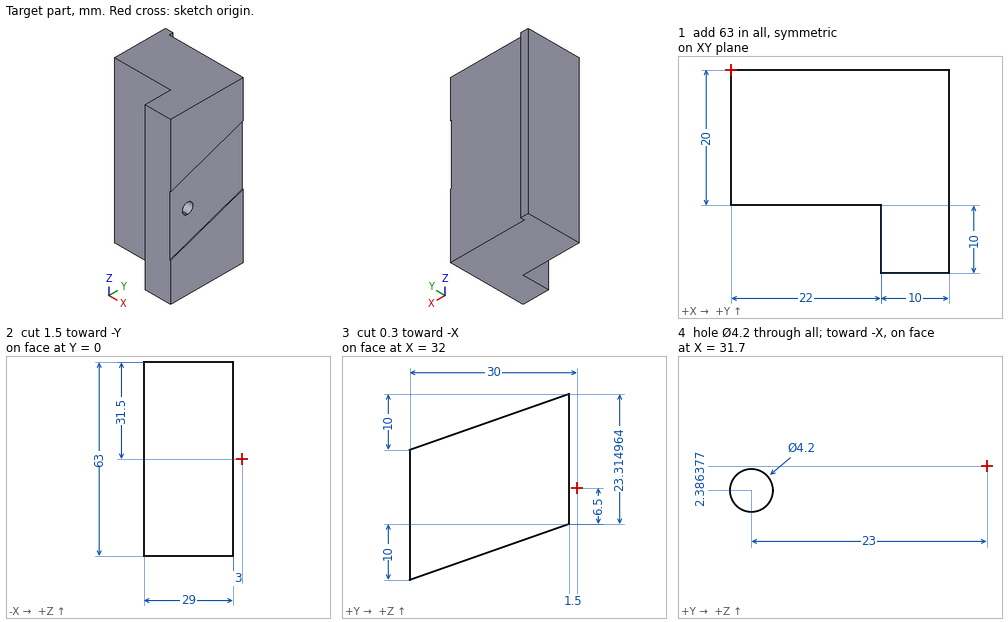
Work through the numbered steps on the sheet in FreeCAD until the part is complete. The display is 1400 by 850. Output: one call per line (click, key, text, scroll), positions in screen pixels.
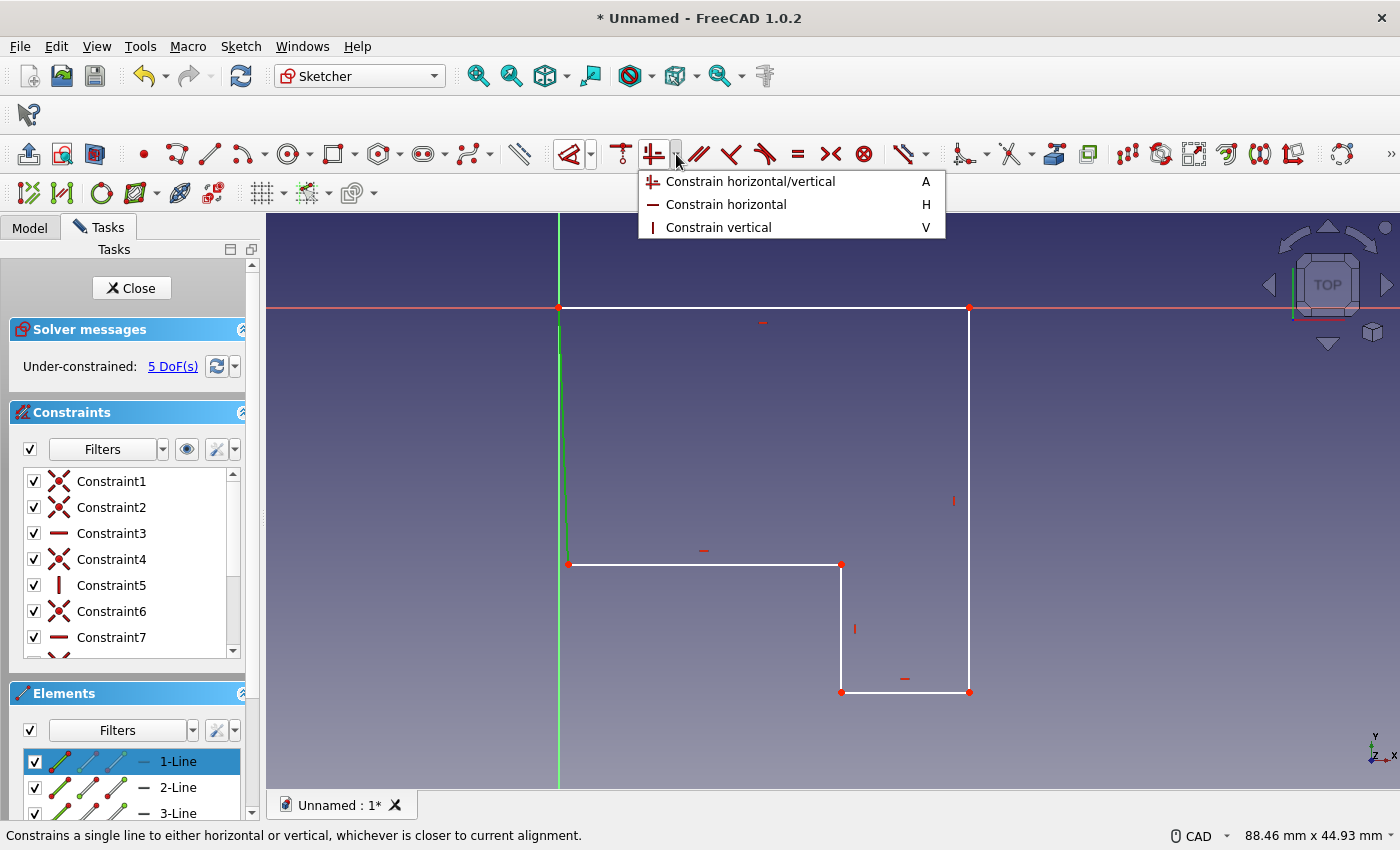
click(792, 228)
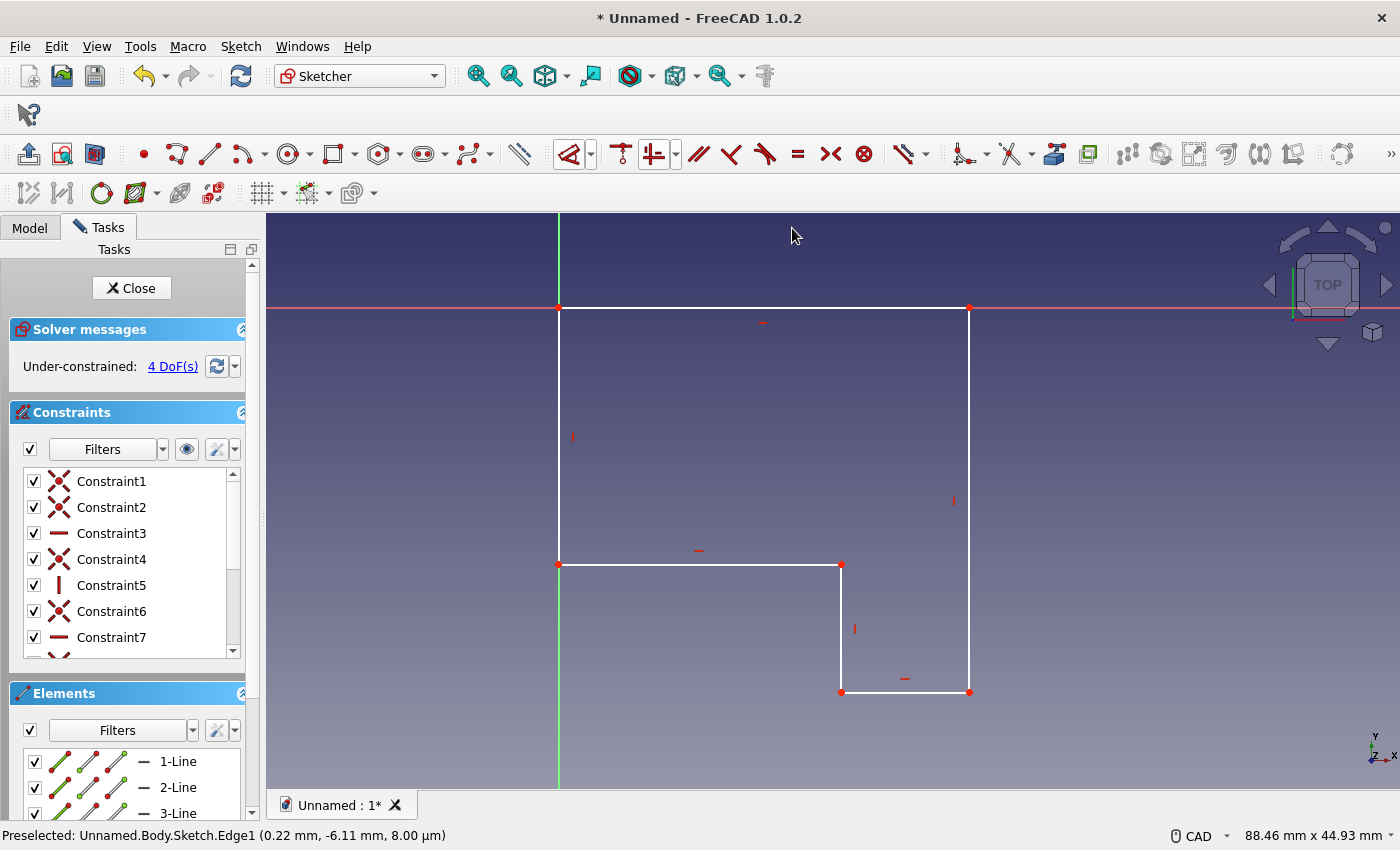
click(568, 154)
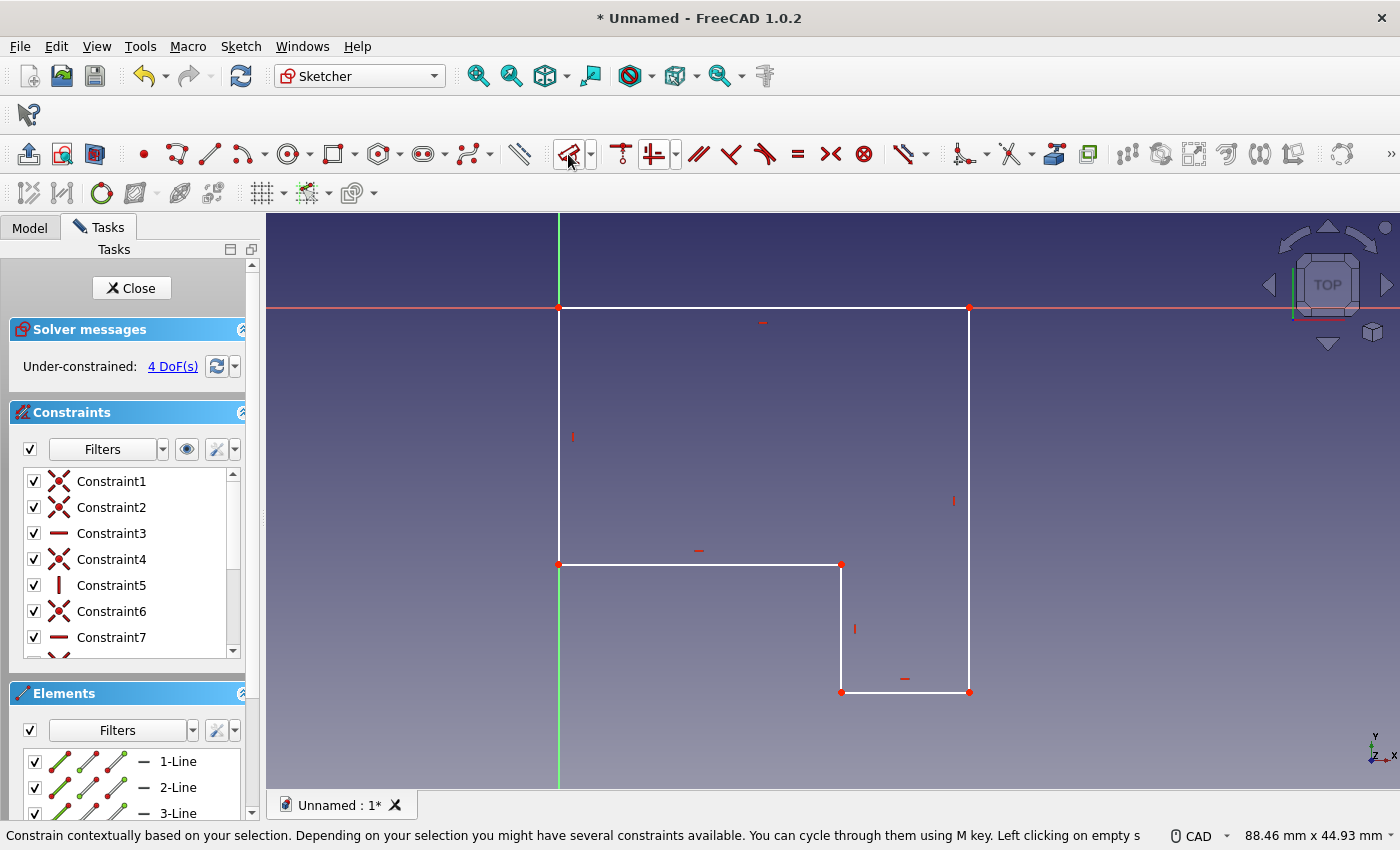
click(559, 385)
click(525, 436)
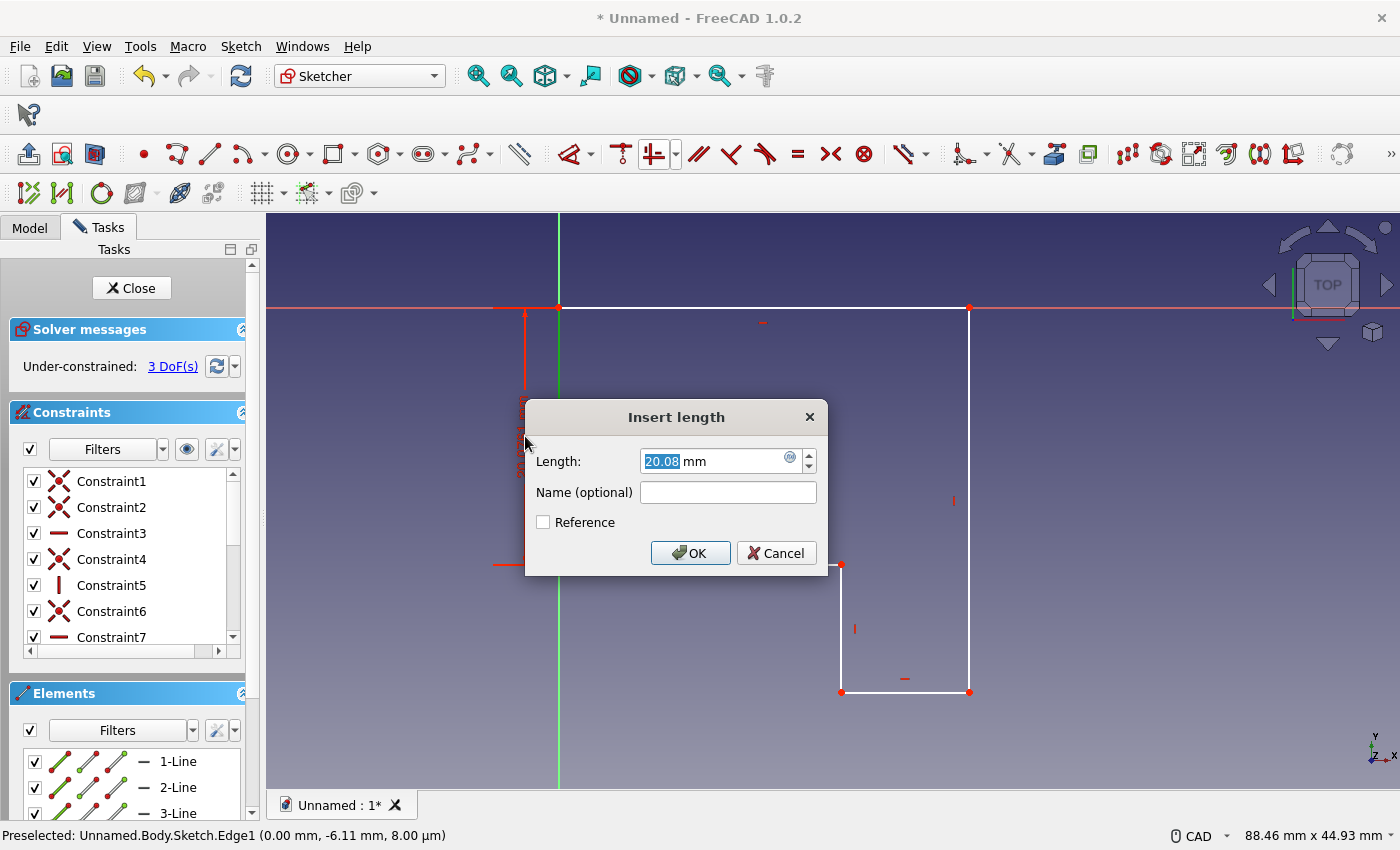
text(20)
key(Return)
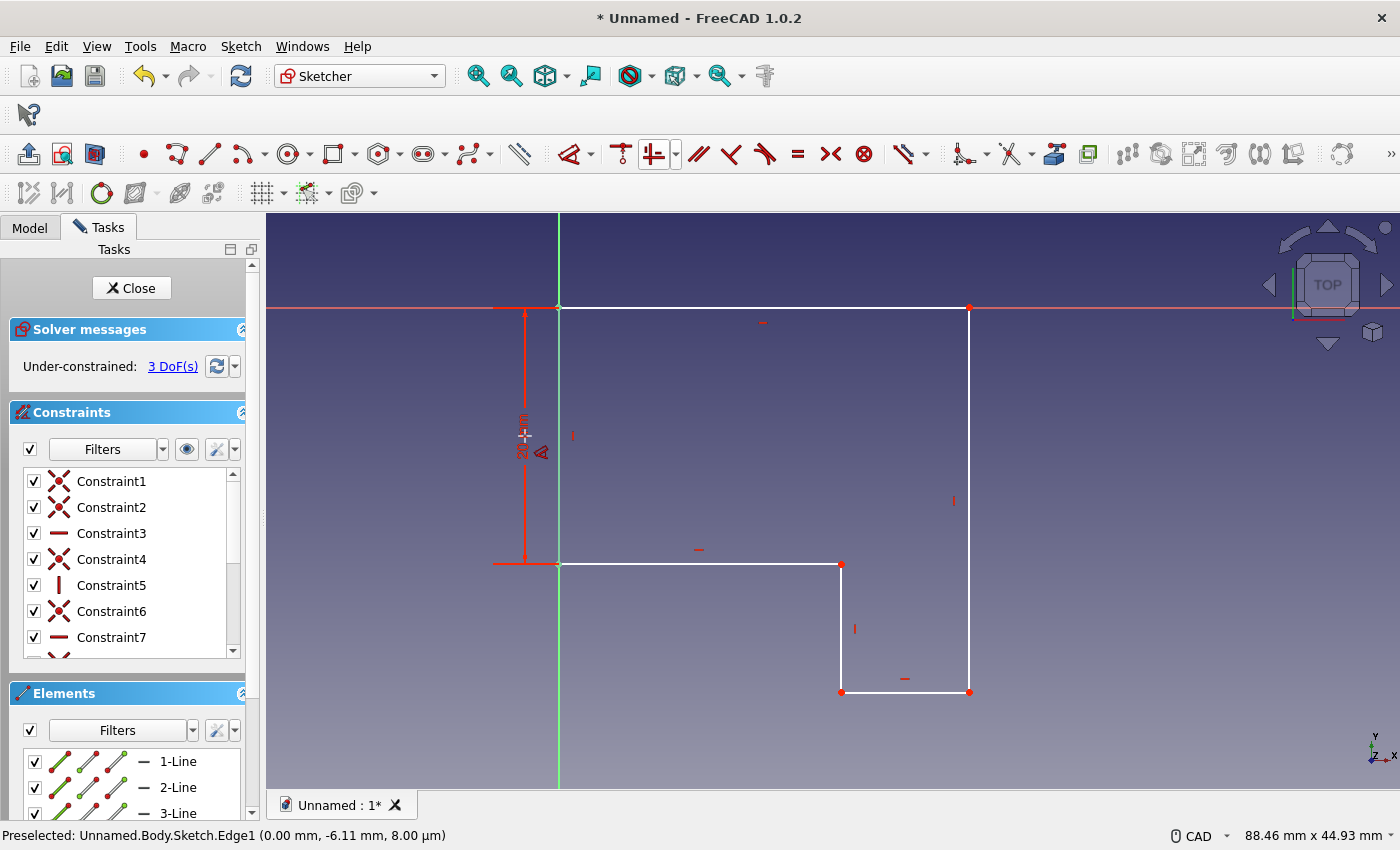
click(643, 564)
click(700, 598)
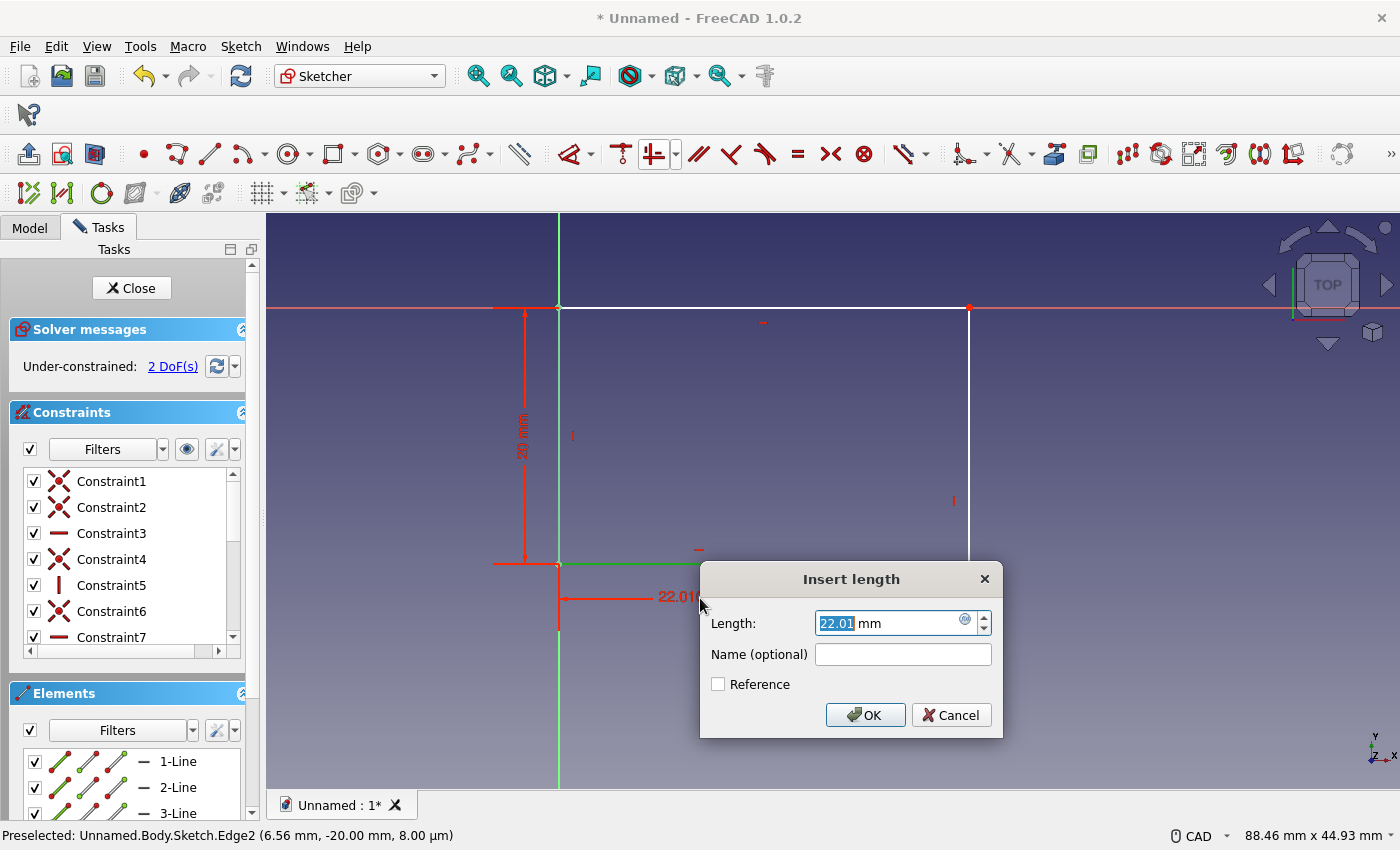
text(22)
key(Return)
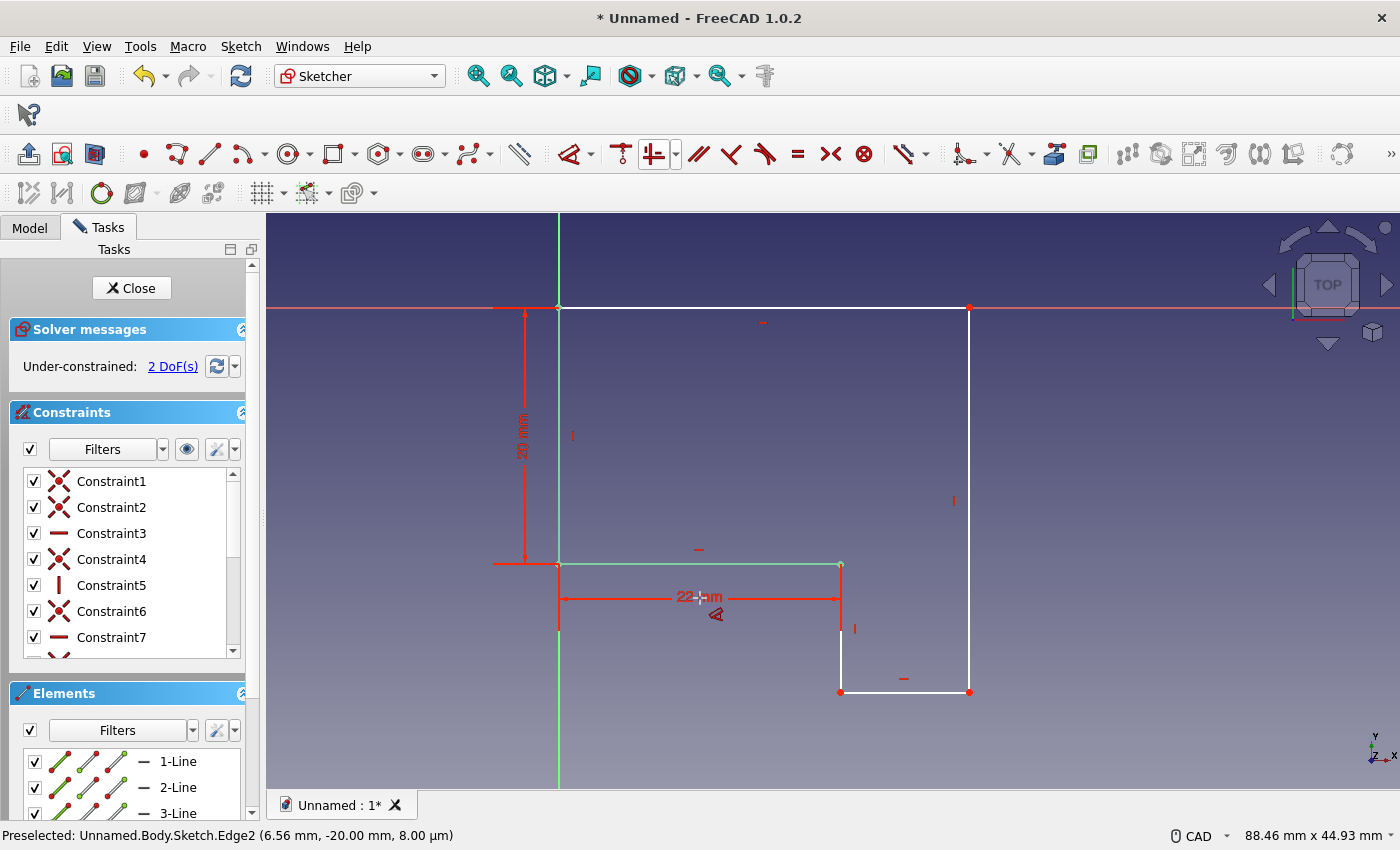
click(841, 603)
click(875, 629)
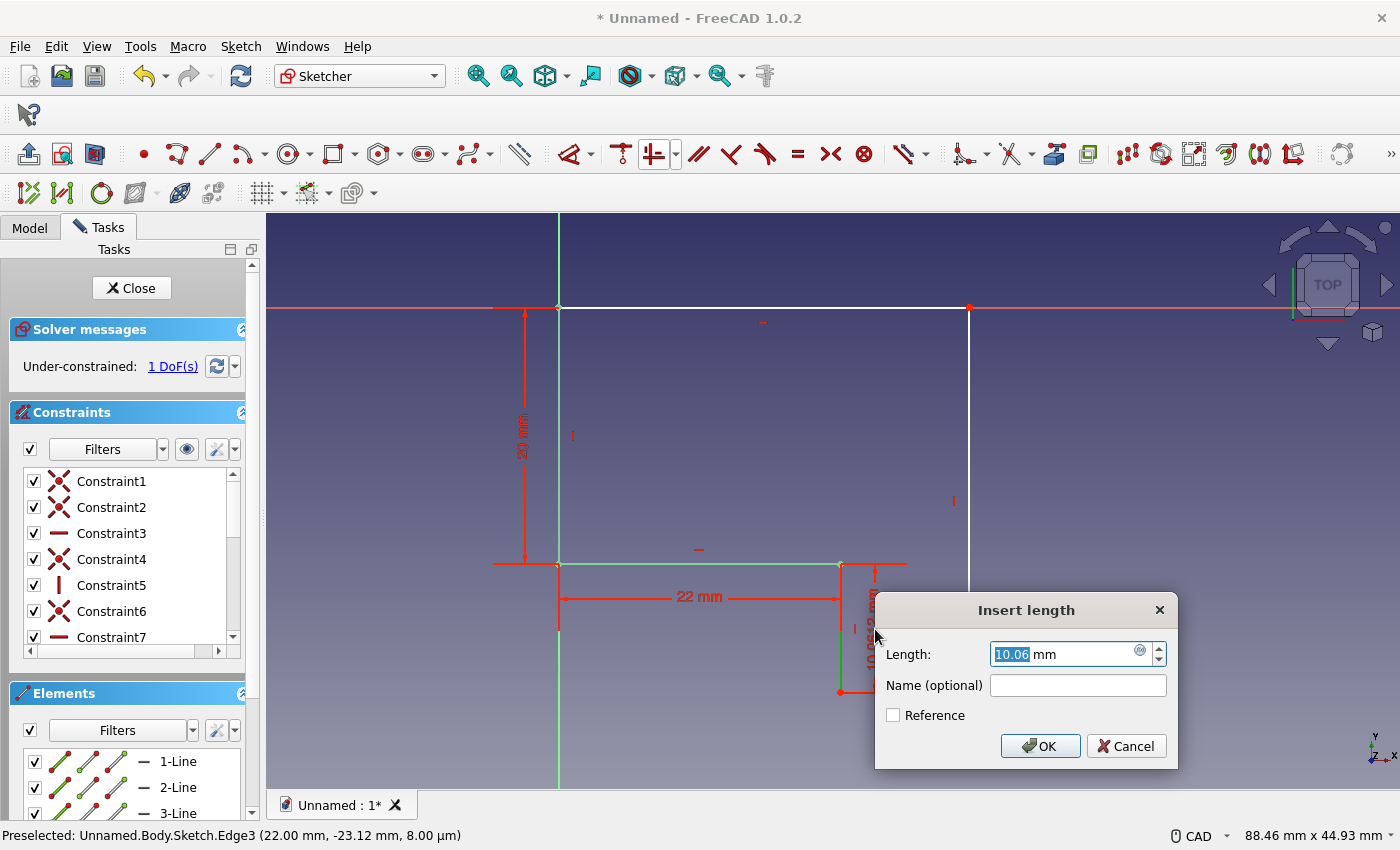
text(10)
key(Return)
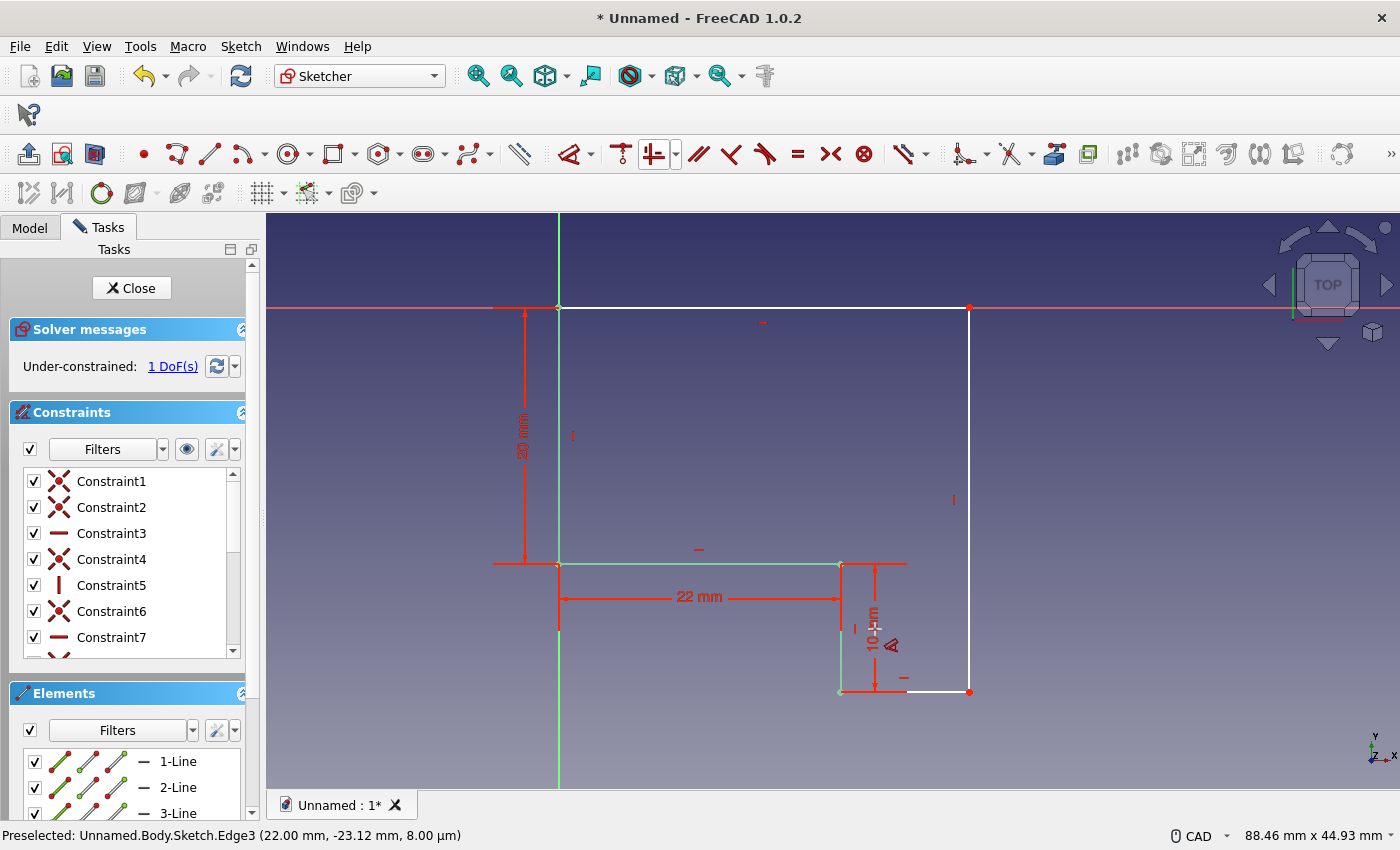
click(879, 692)
click(905, 726)